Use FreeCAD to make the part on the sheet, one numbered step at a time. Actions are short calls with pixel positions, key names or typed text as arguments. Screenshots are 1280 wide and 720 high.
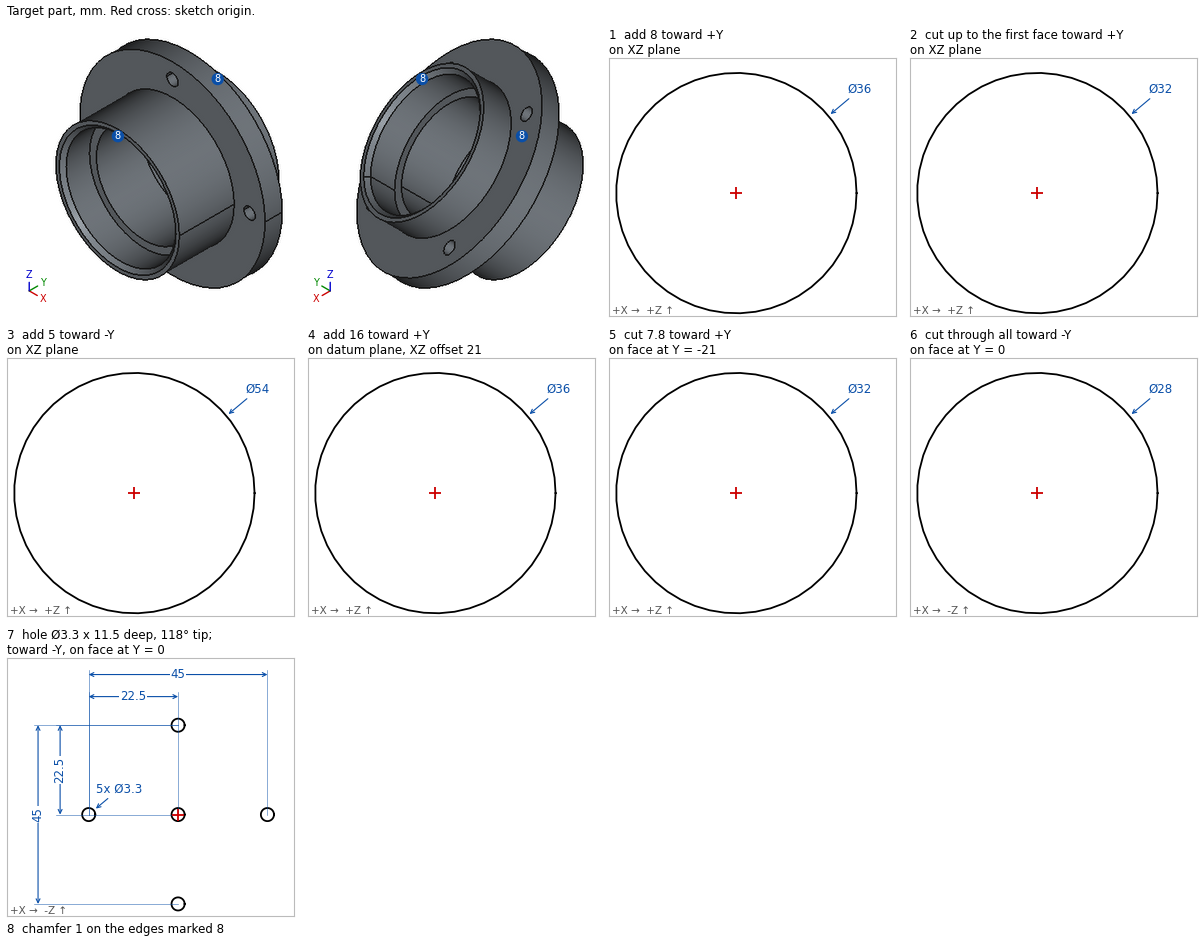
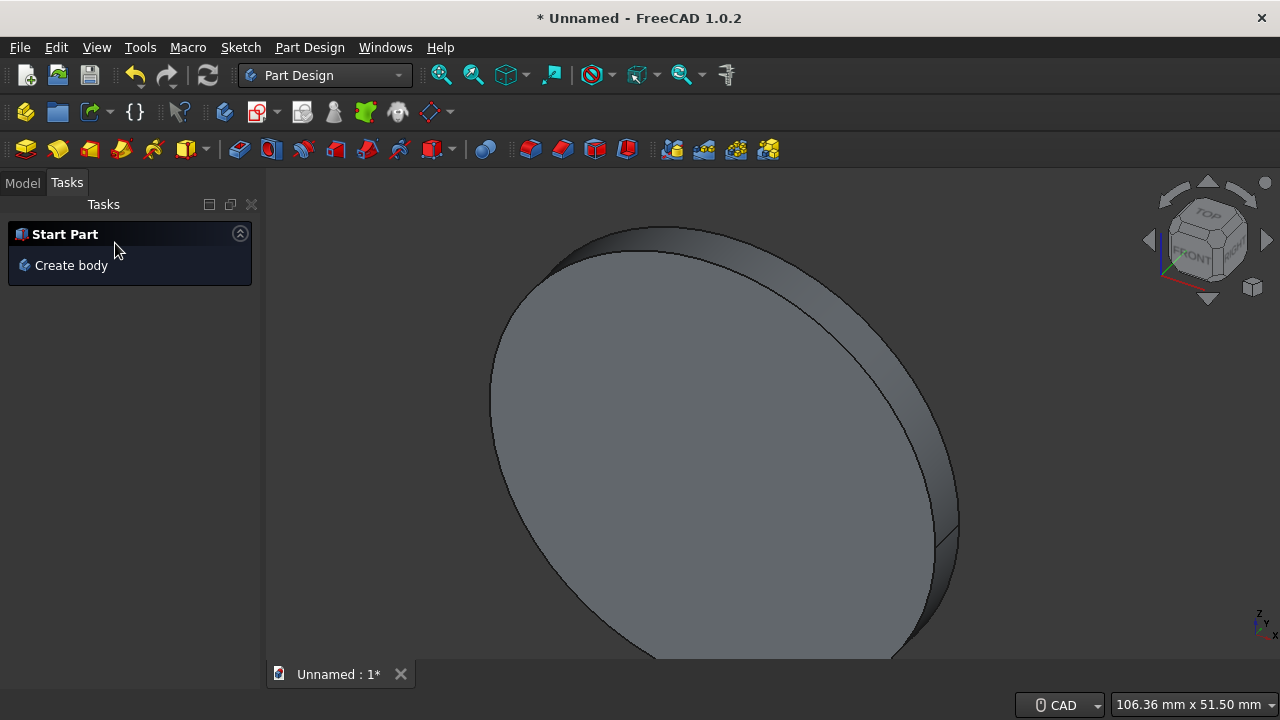
click(442, 76)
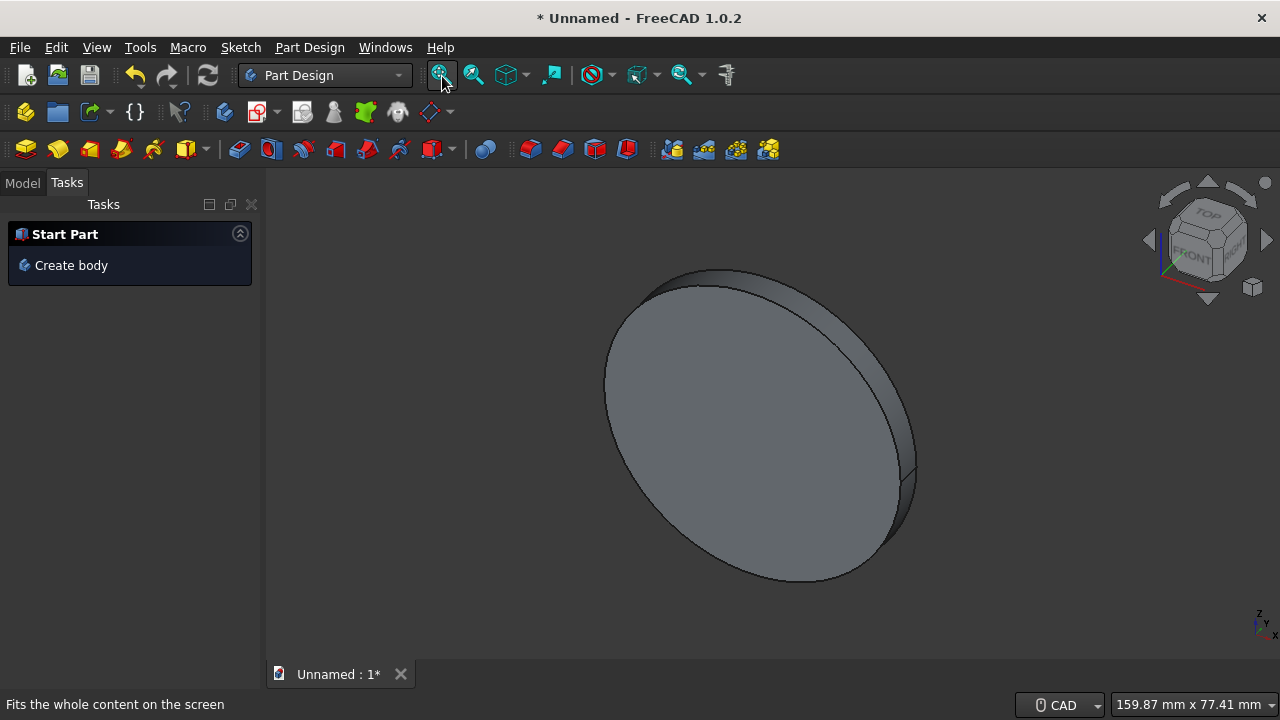
click(23, 182)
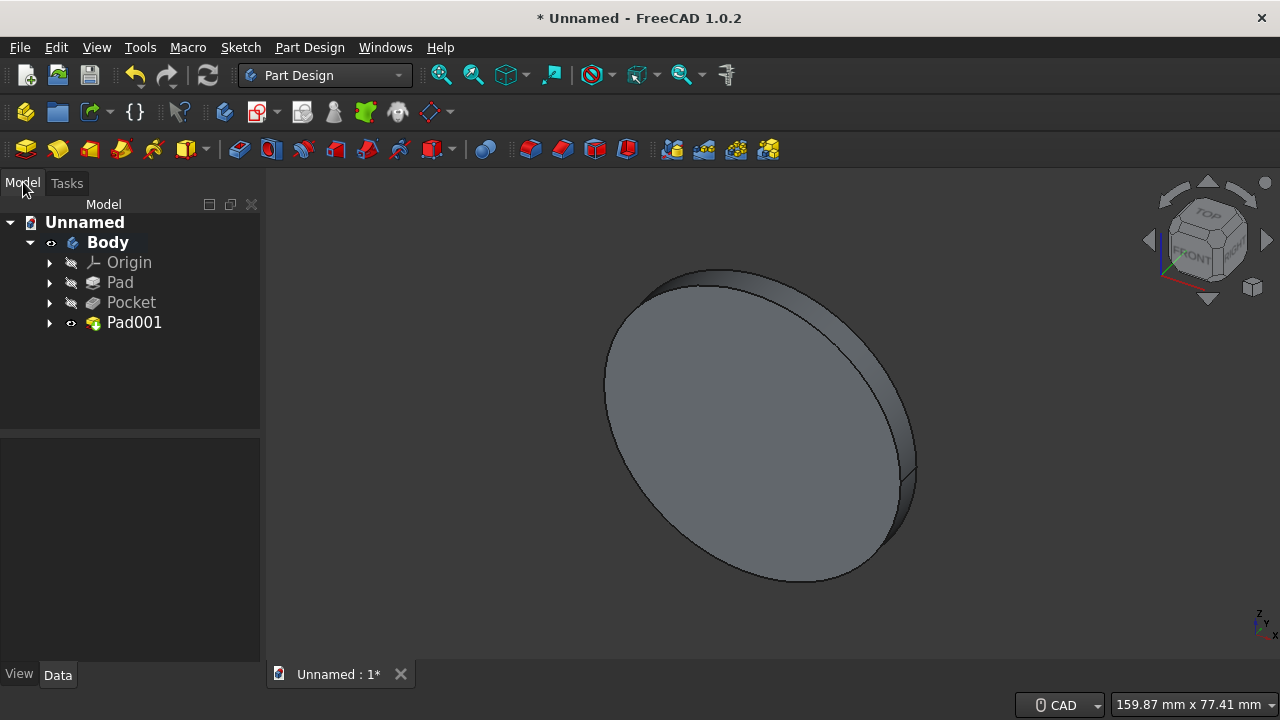
click(50, 263)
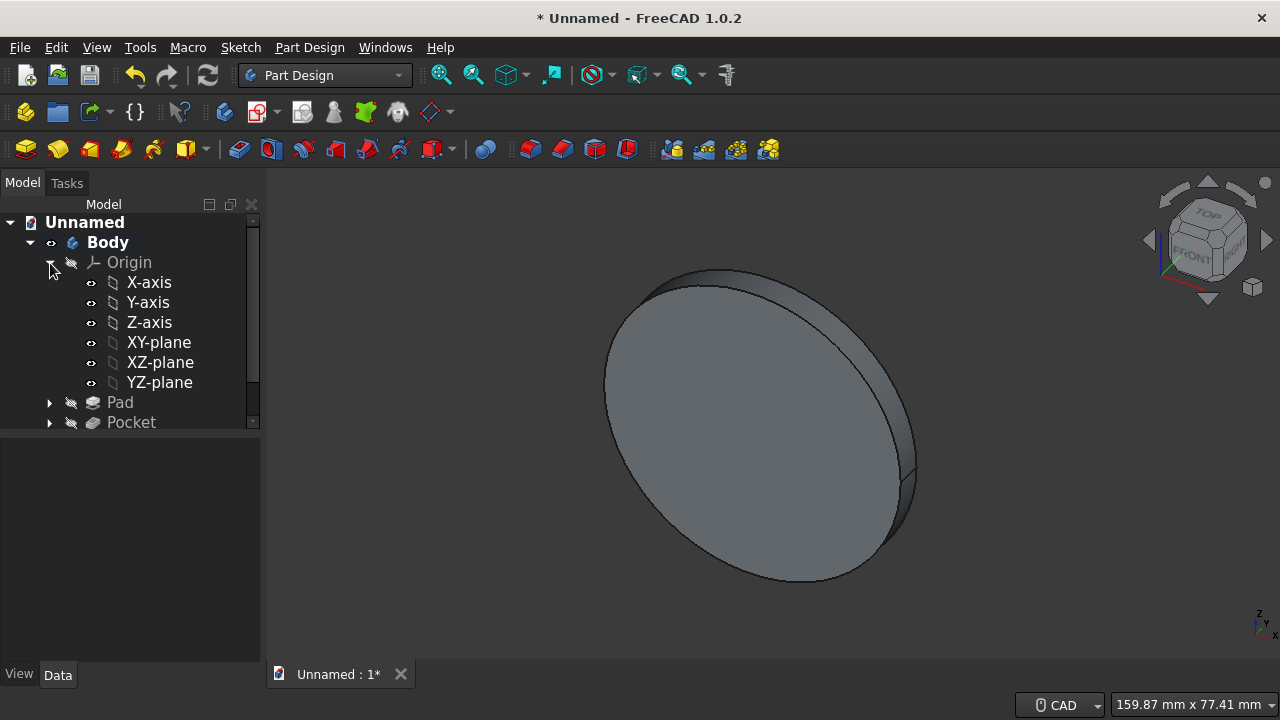
click(136, 363)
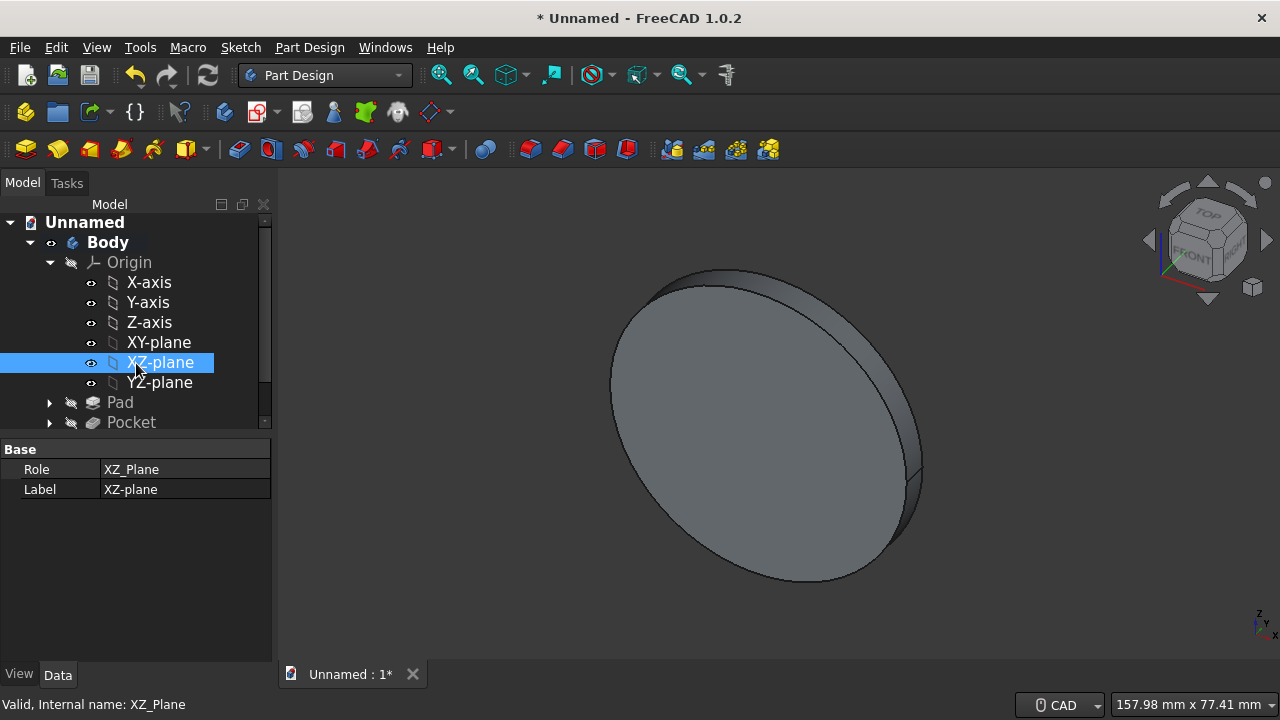
click(430, 112)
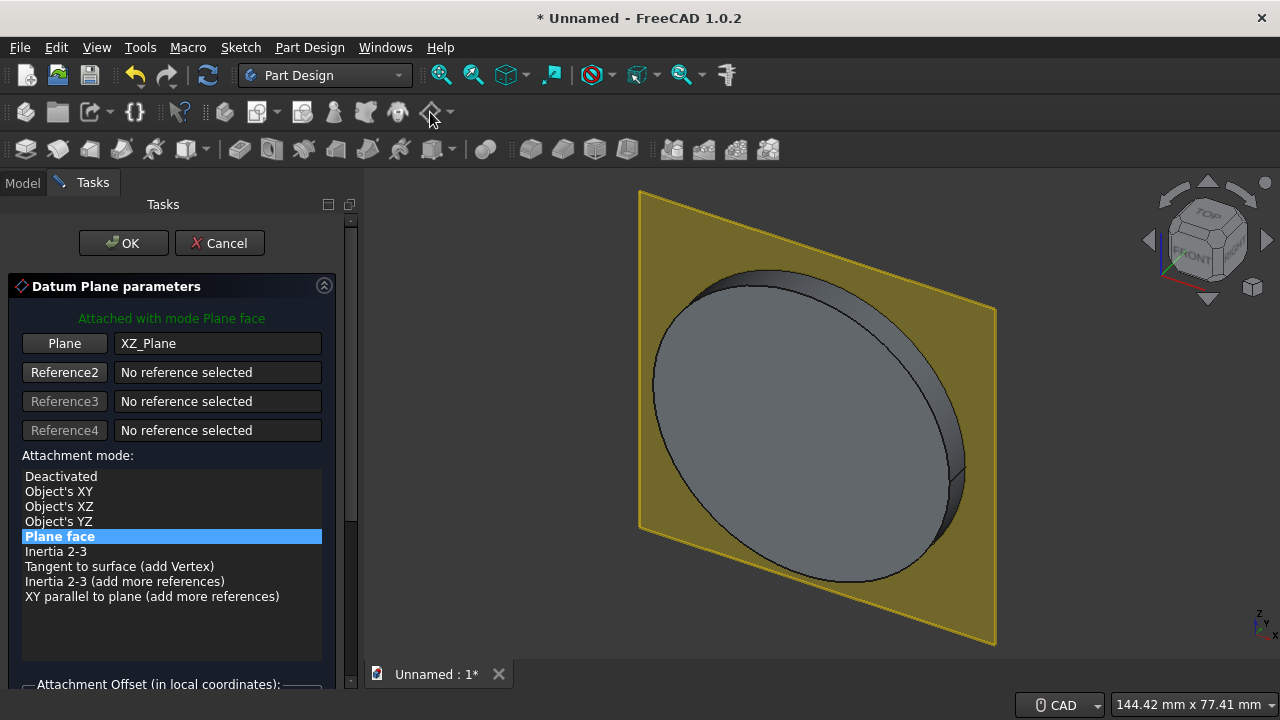
scroll(351, 451, down, 3)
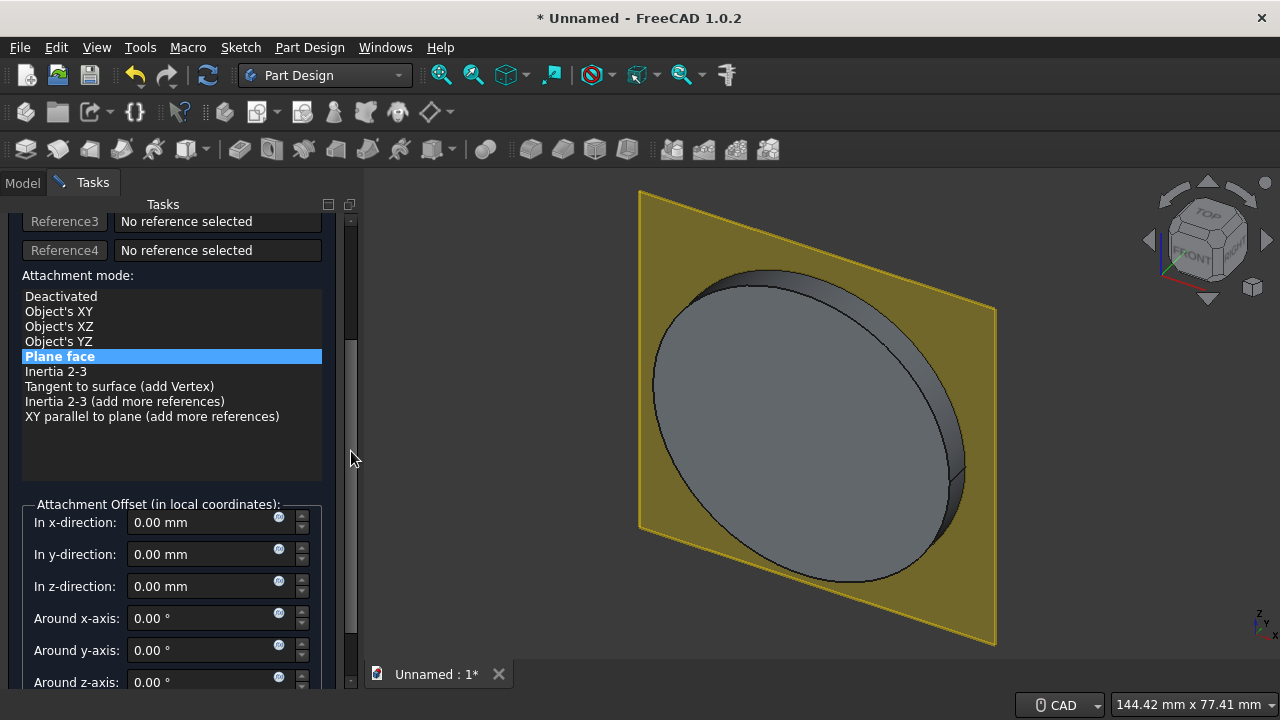
triple_click(210, 586)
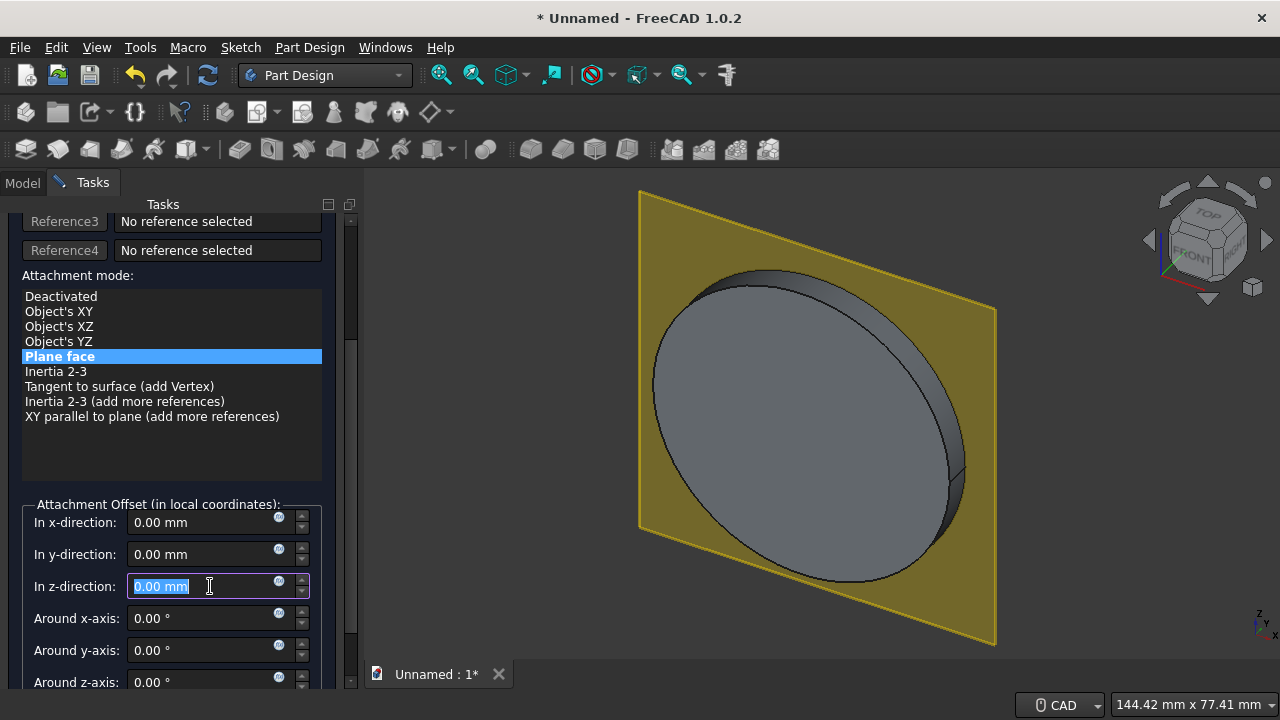
text(21)
key(Tab)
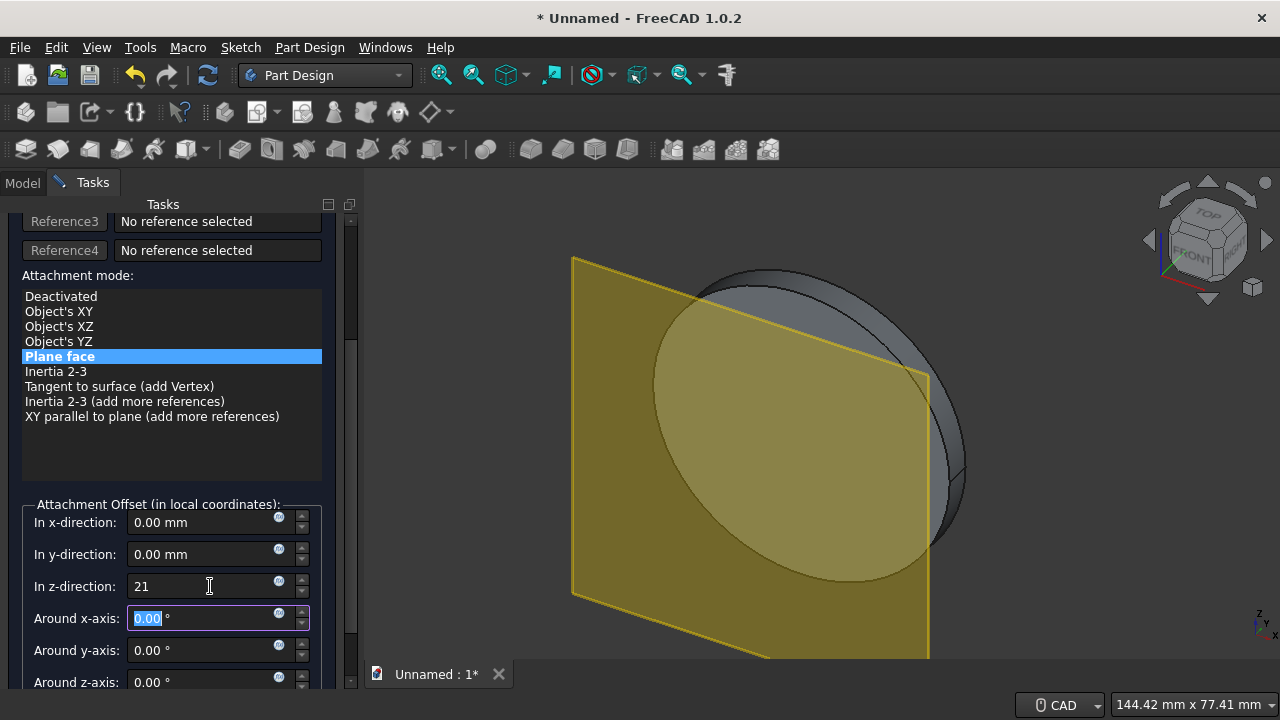
scroll(351, 451, up, 4)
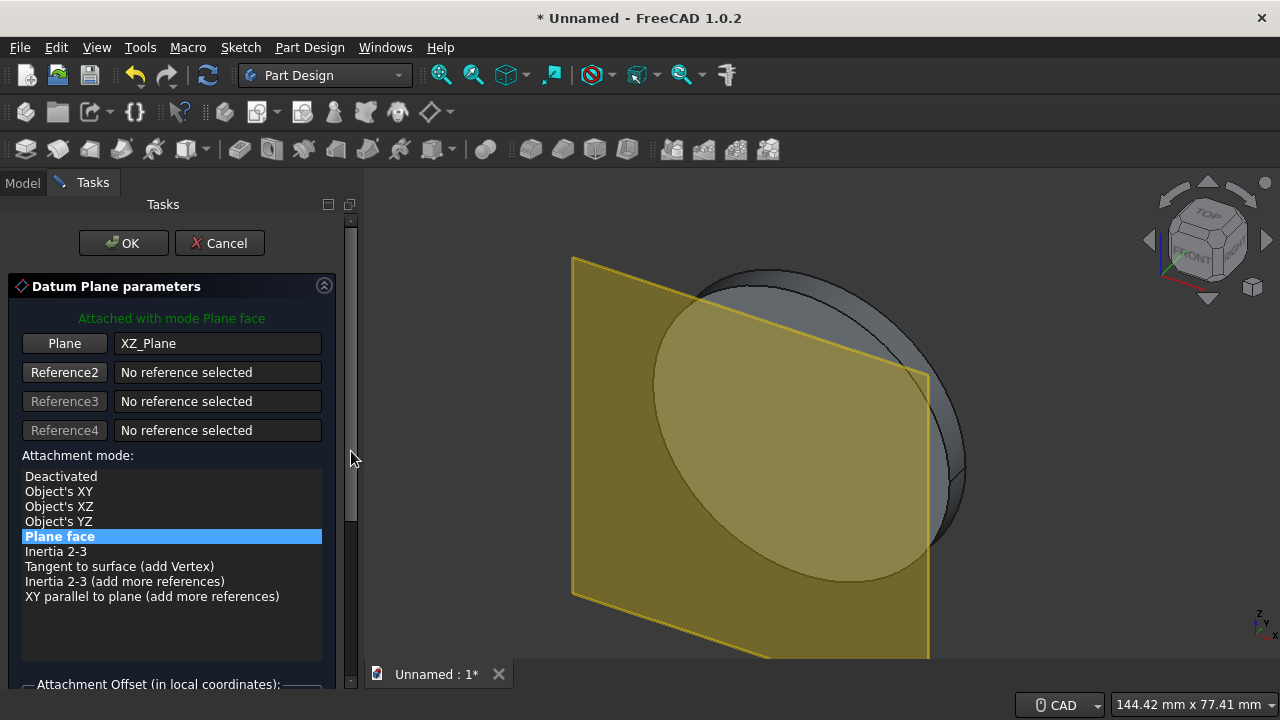
click(124, 243)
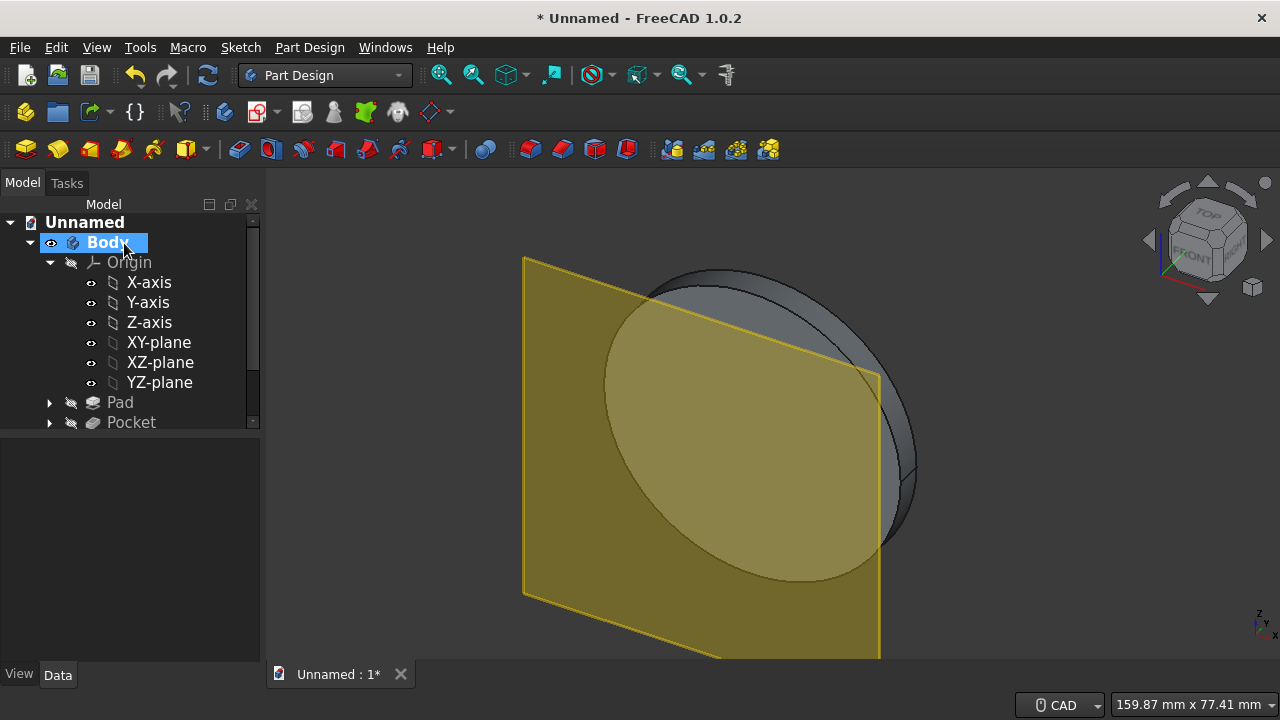
scroll(100, 318, down, 3)